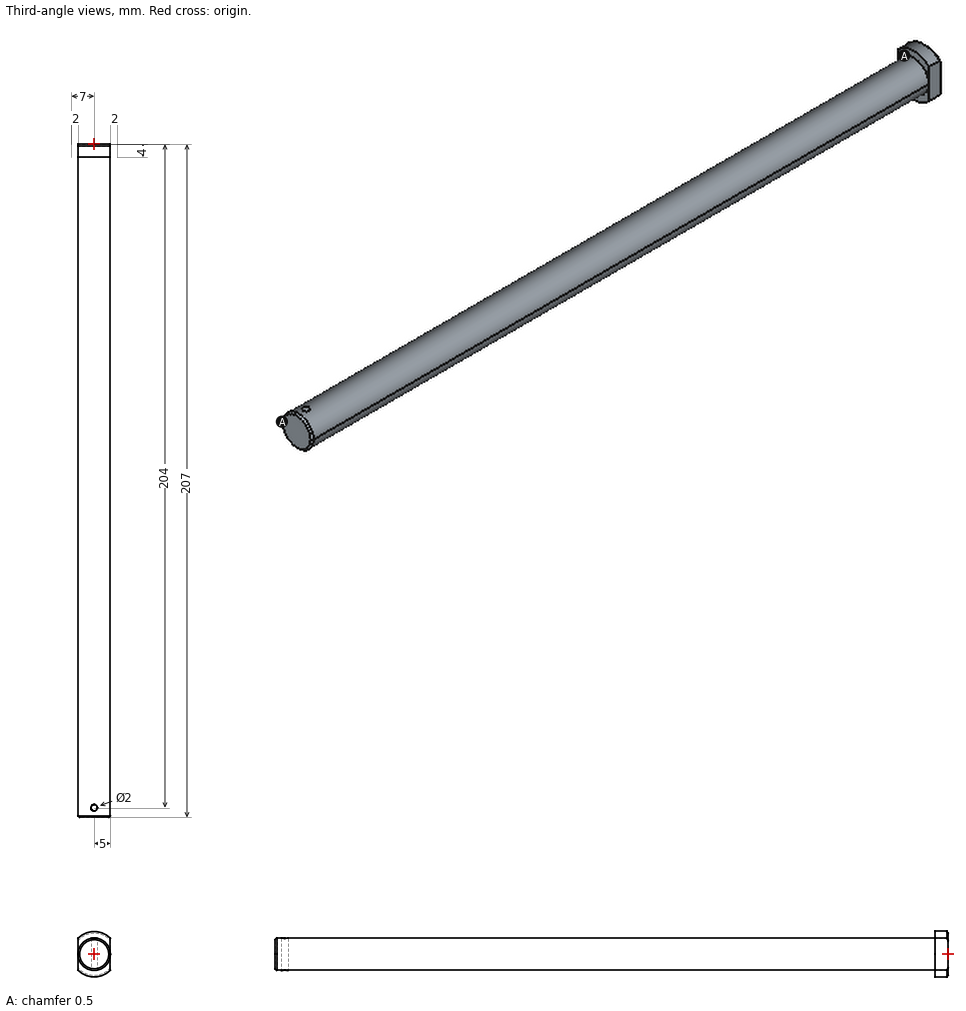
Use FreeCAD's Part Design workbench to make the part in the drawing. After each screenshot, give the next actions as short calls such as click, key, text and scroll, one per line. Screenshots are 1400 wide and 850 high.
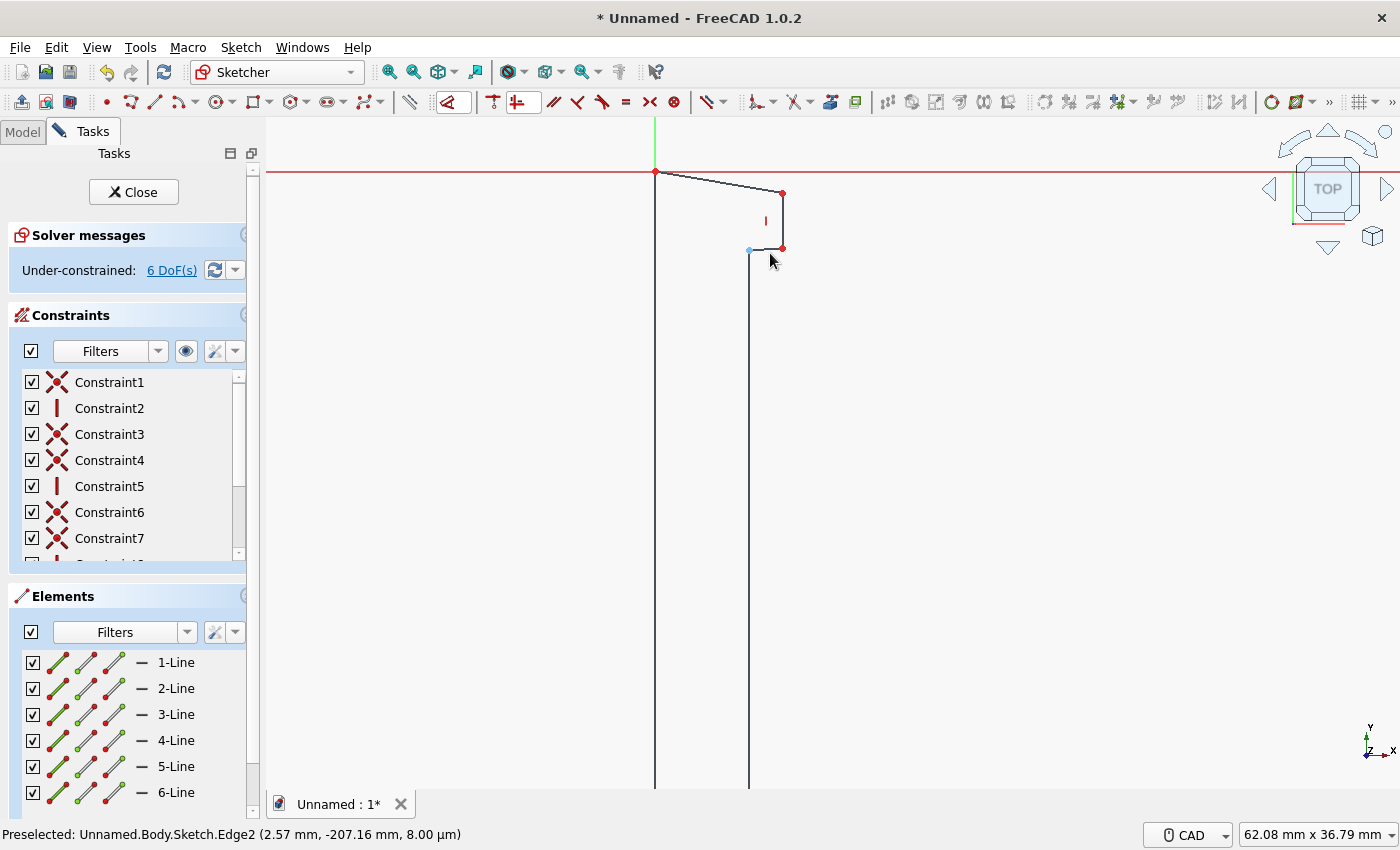
click(766, 249)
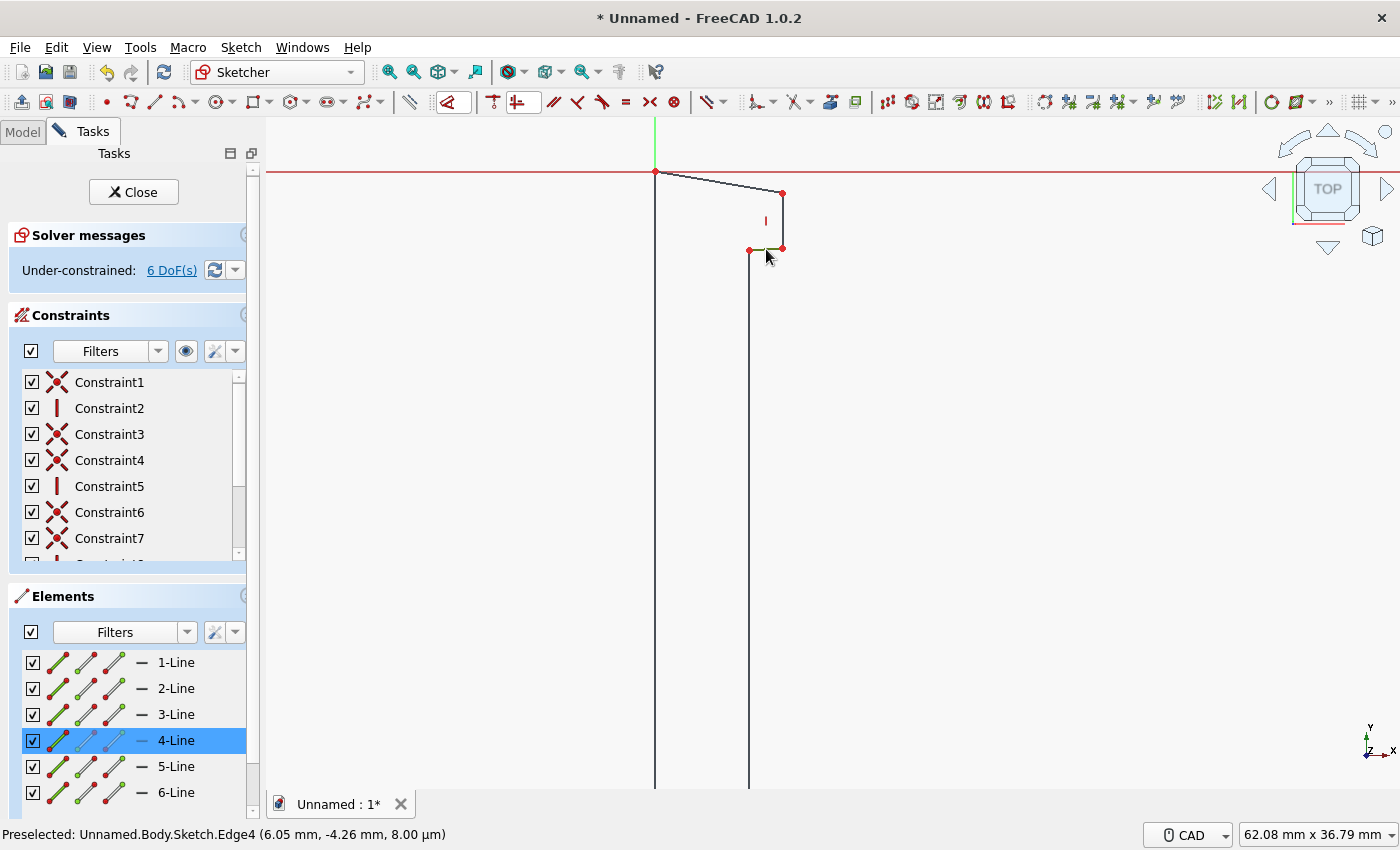
key(h)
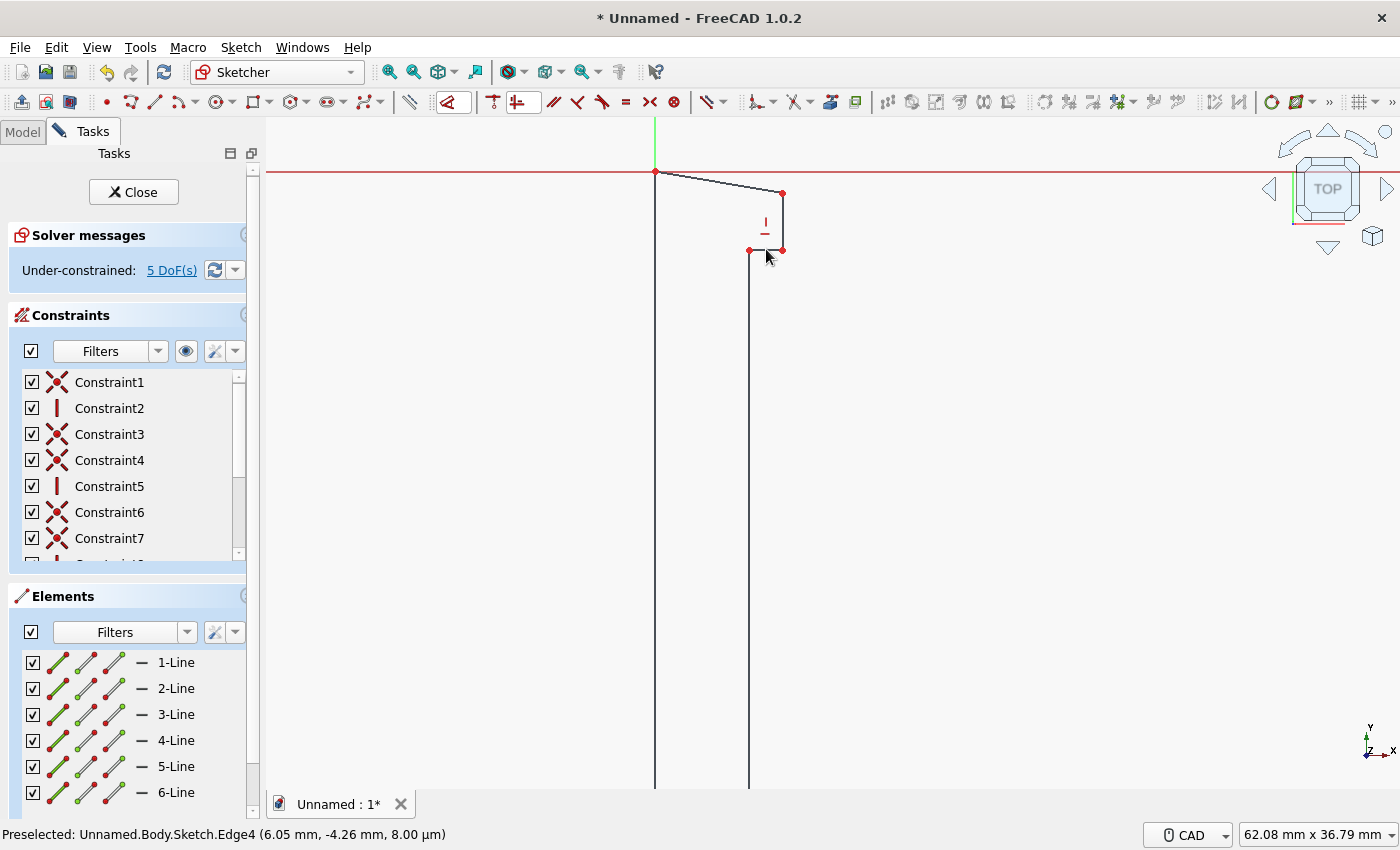
click(745, 187)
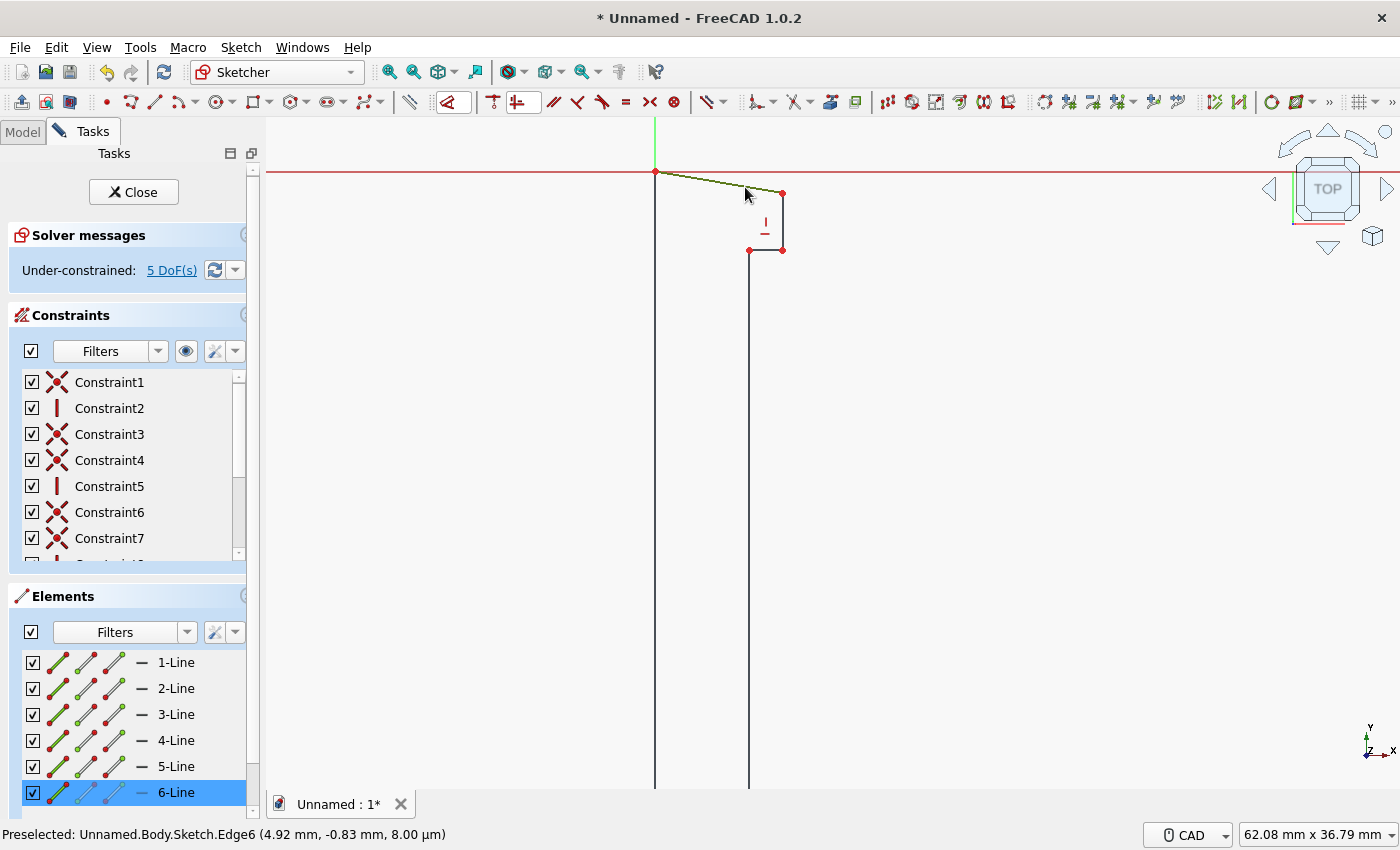
key(h)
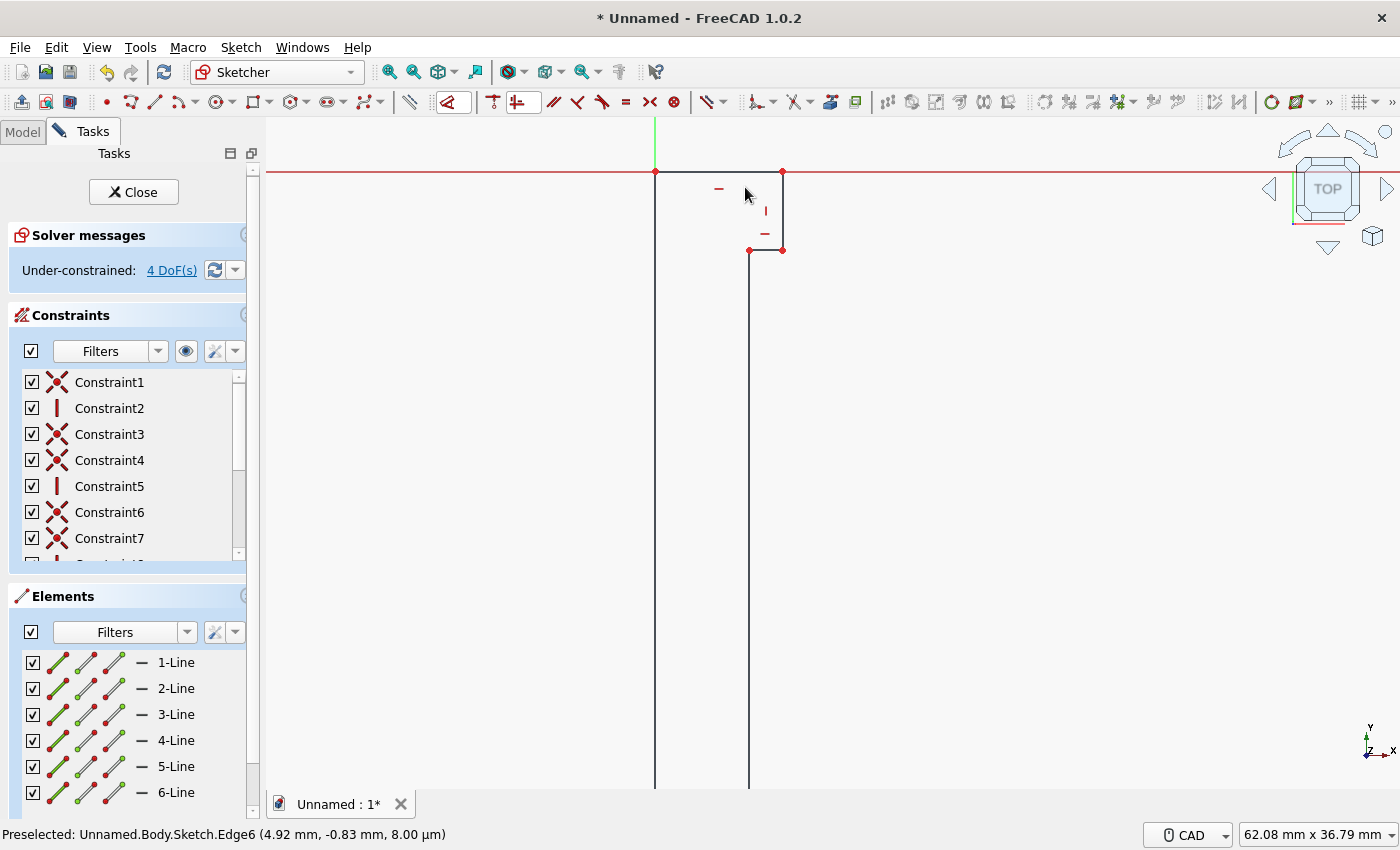
click(448, 102)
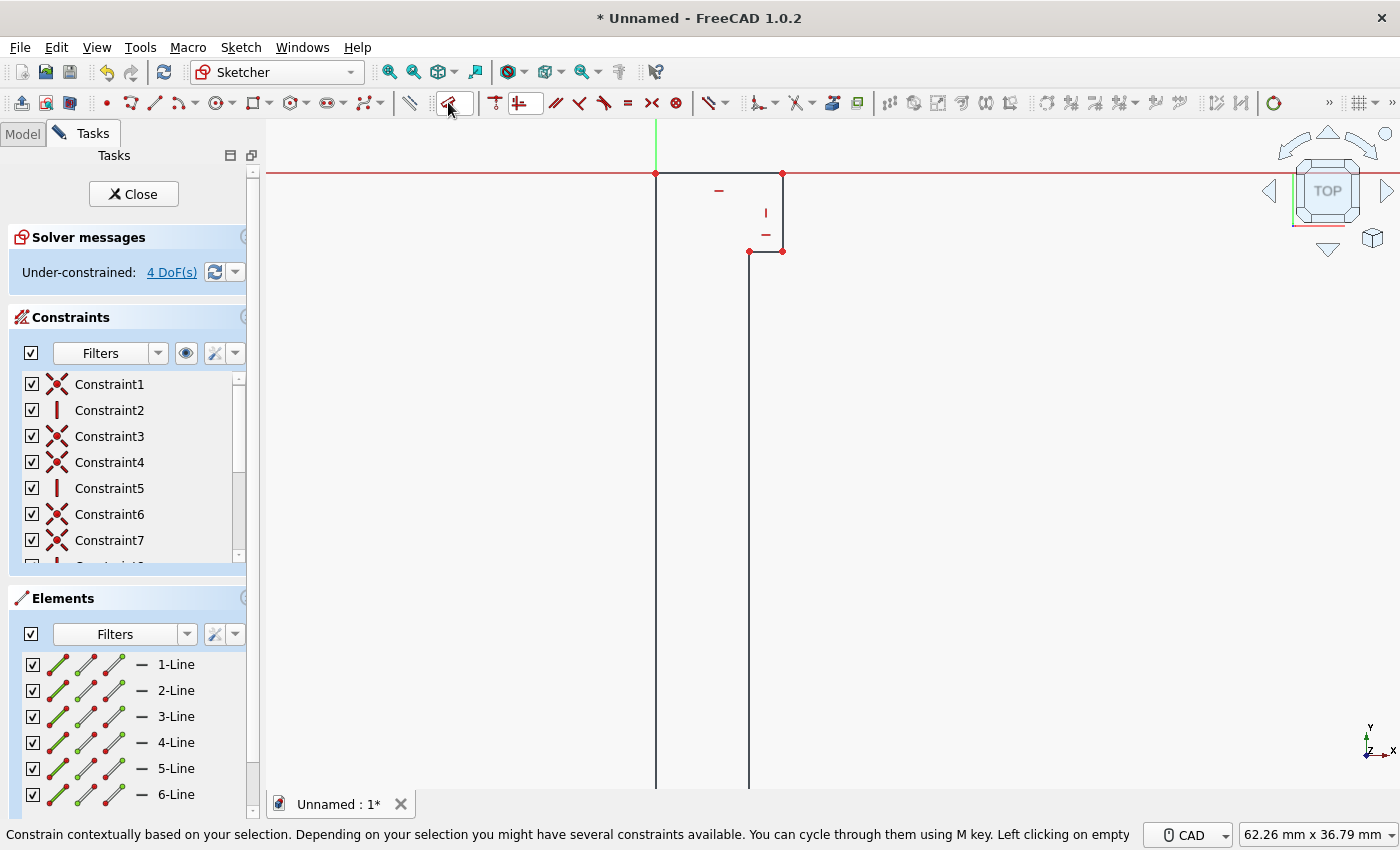
scroll(770, 254, down, 11)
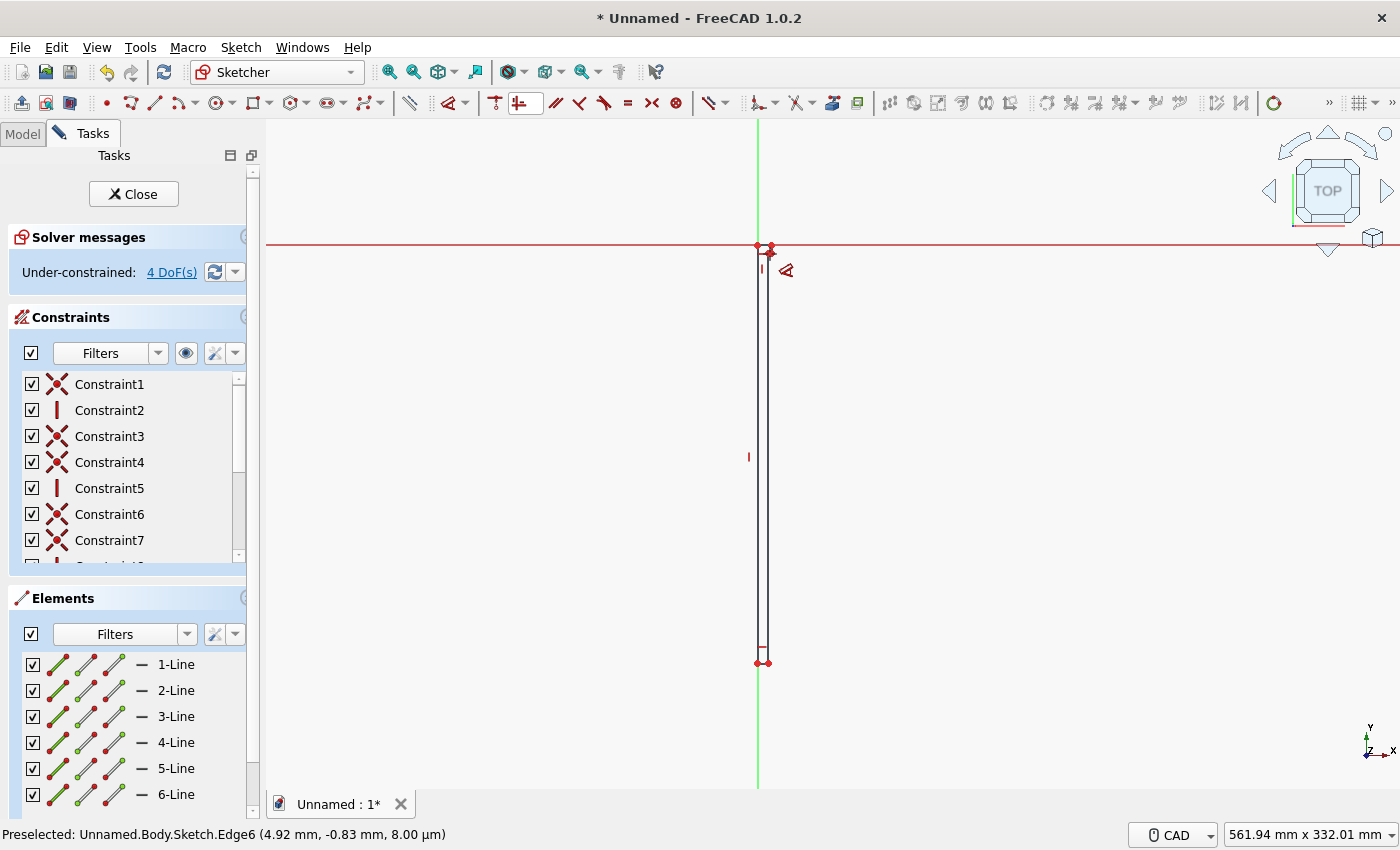
scroll(761, 664, up, 8)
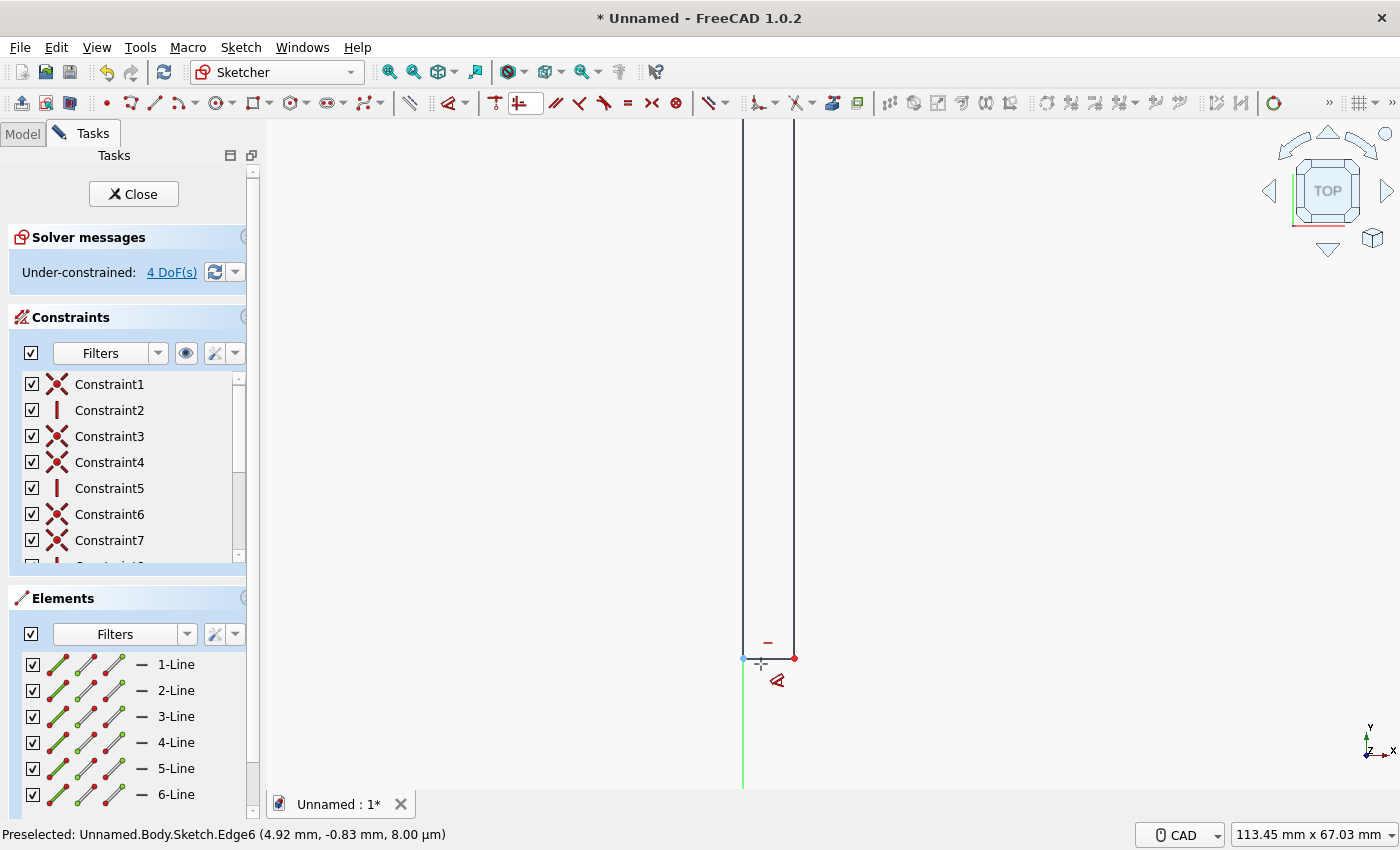
click(759, 659)
click(769, 693)